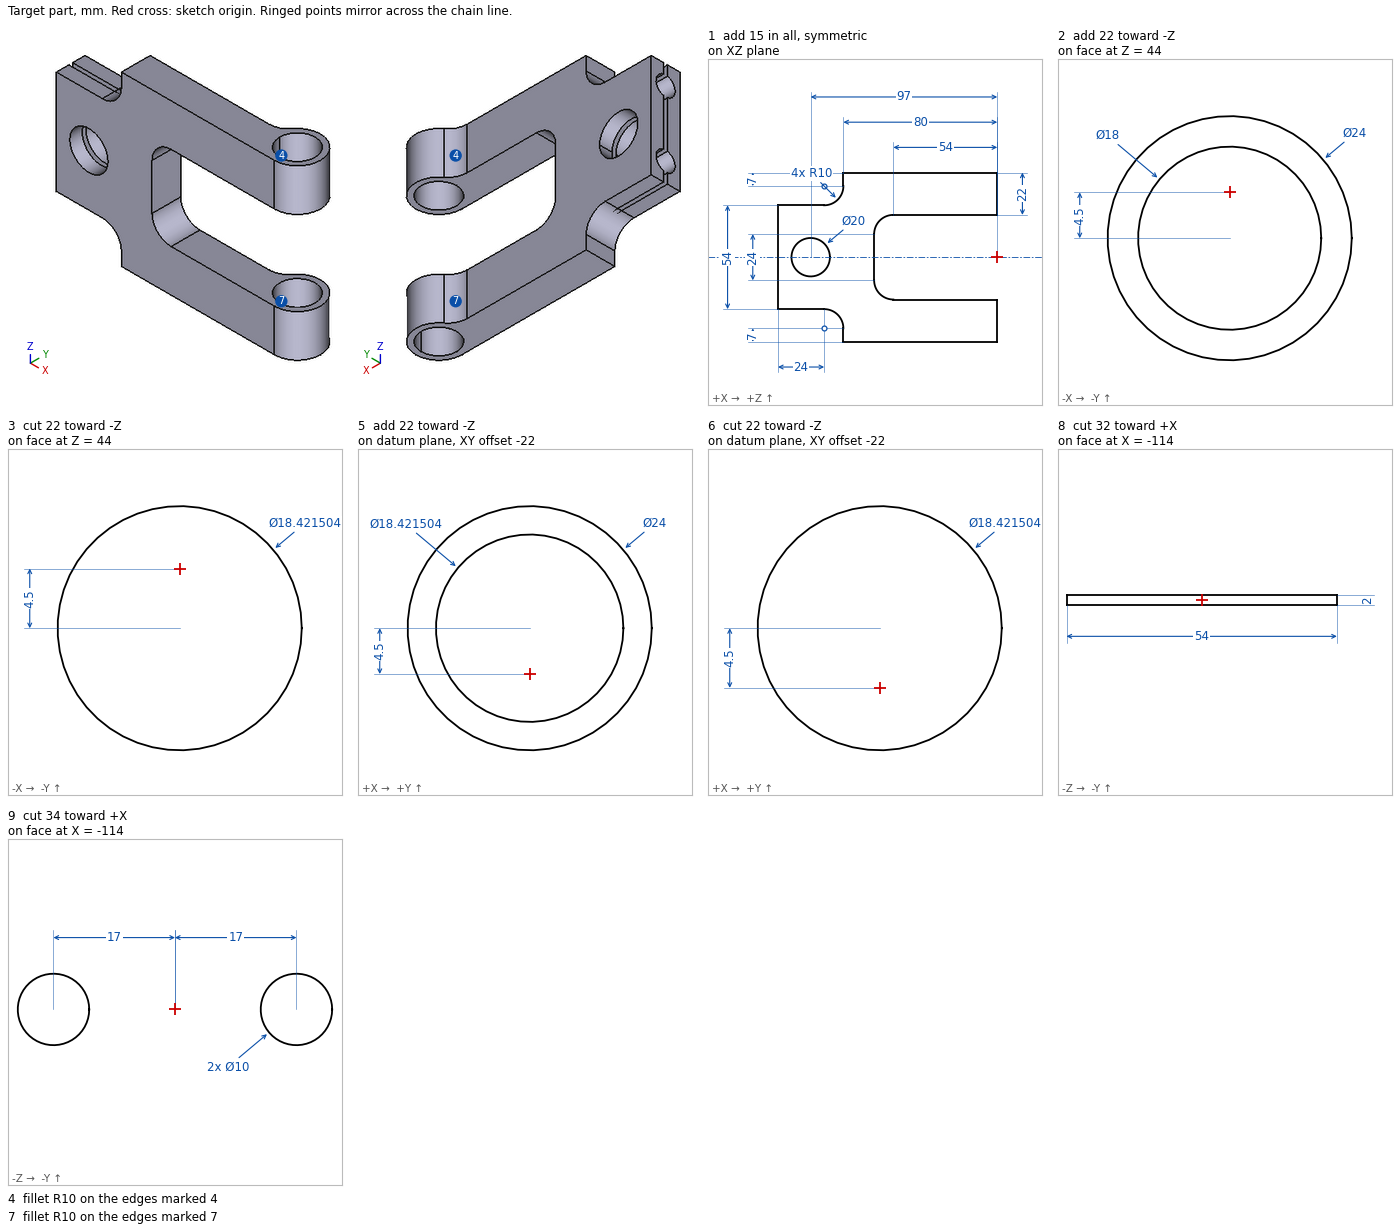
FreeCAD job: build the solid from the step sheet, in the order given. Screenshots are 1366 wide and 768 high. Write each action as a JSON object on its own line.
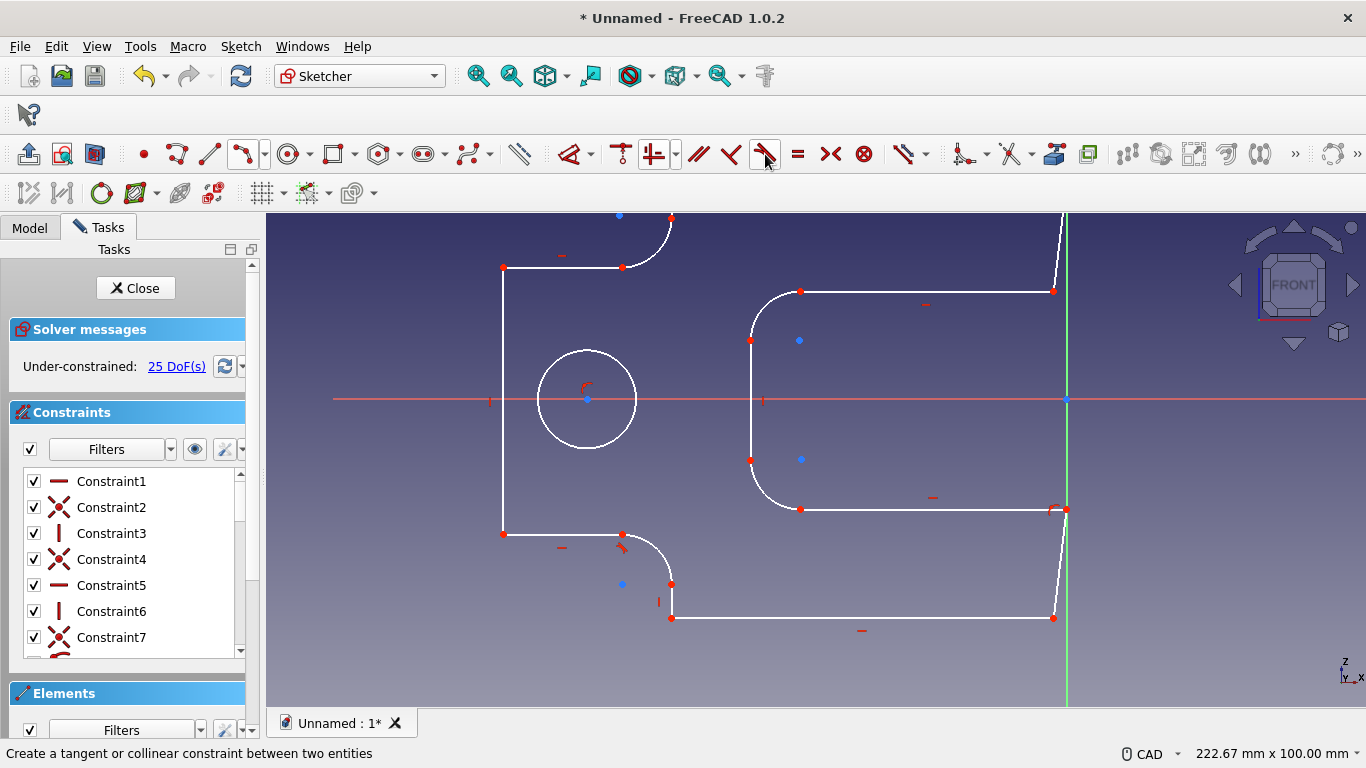
{"action": "left_click", "coordinate": [539, 268]}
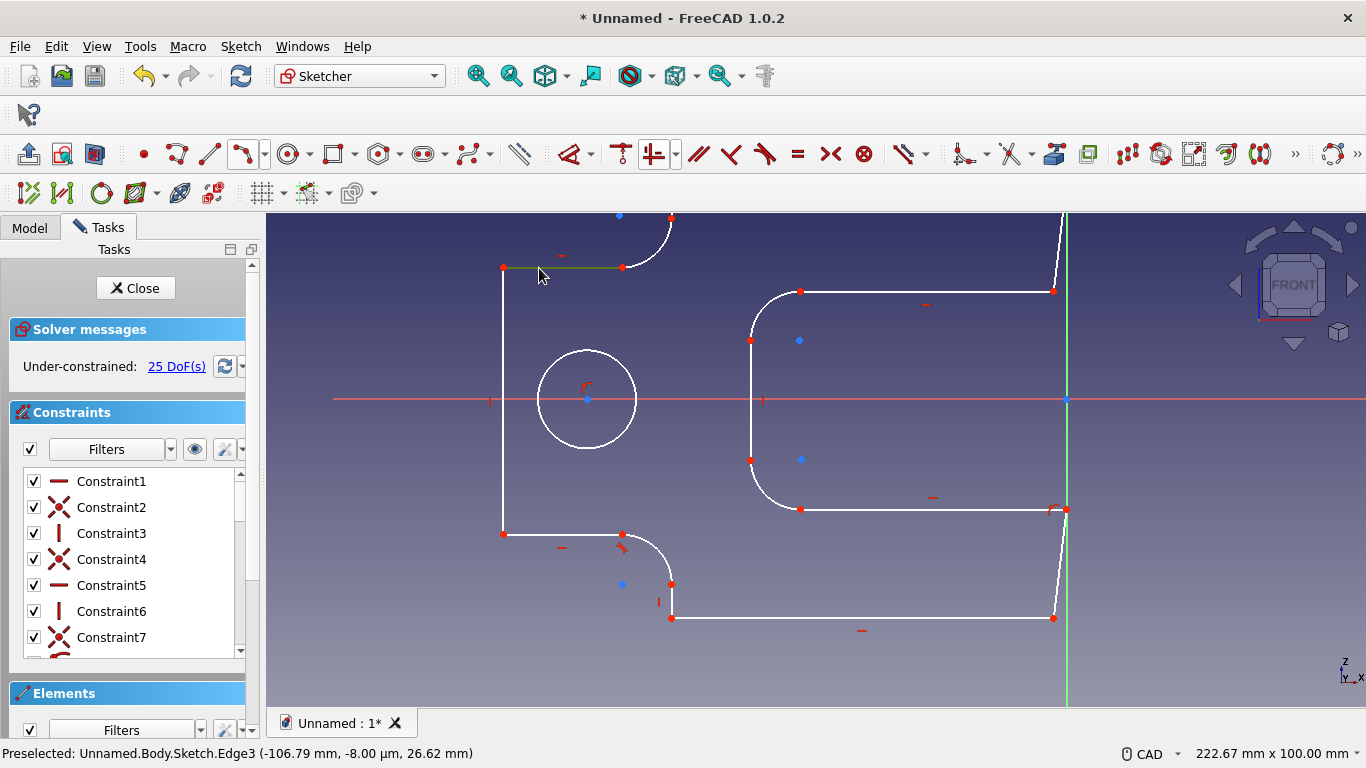
{"action": "left_click", "coordinate": [644, 262]}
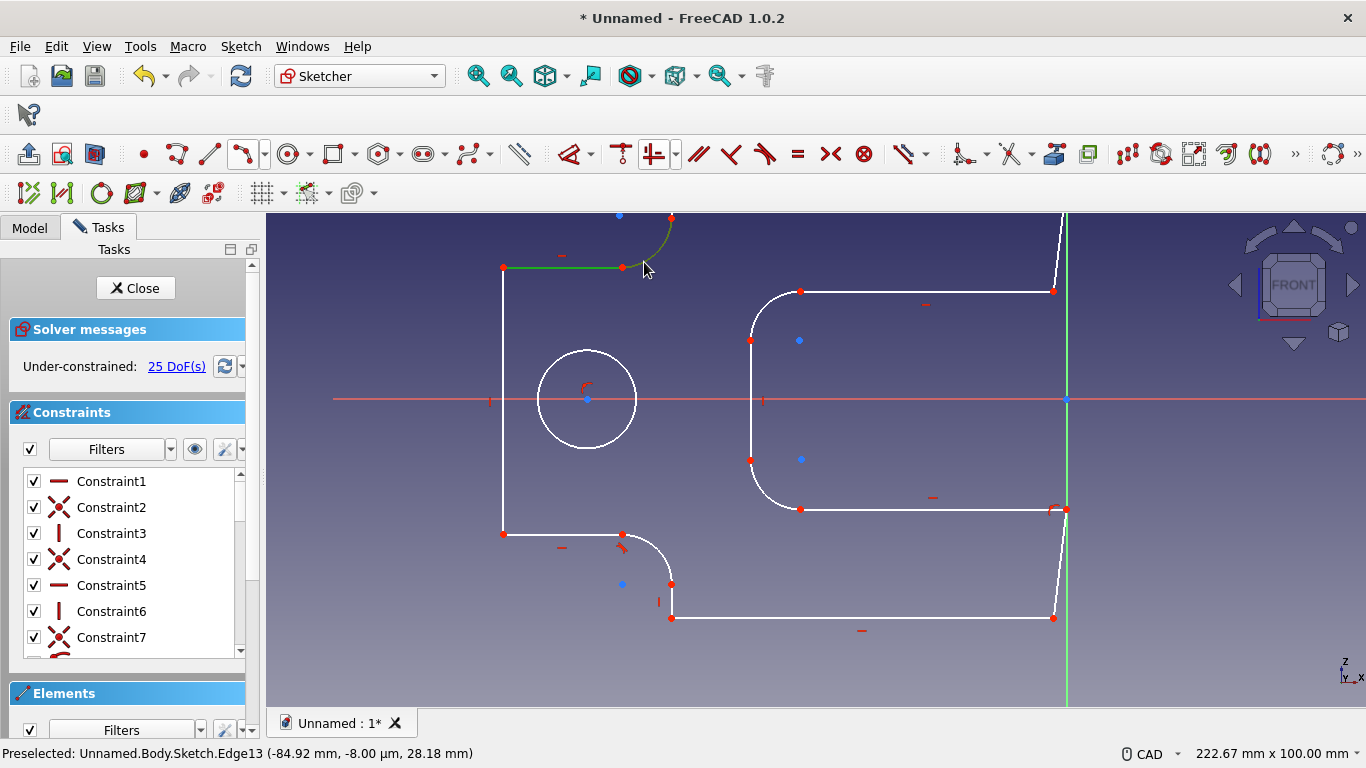
{"action": "left_click", "coordinate": [765, 154]}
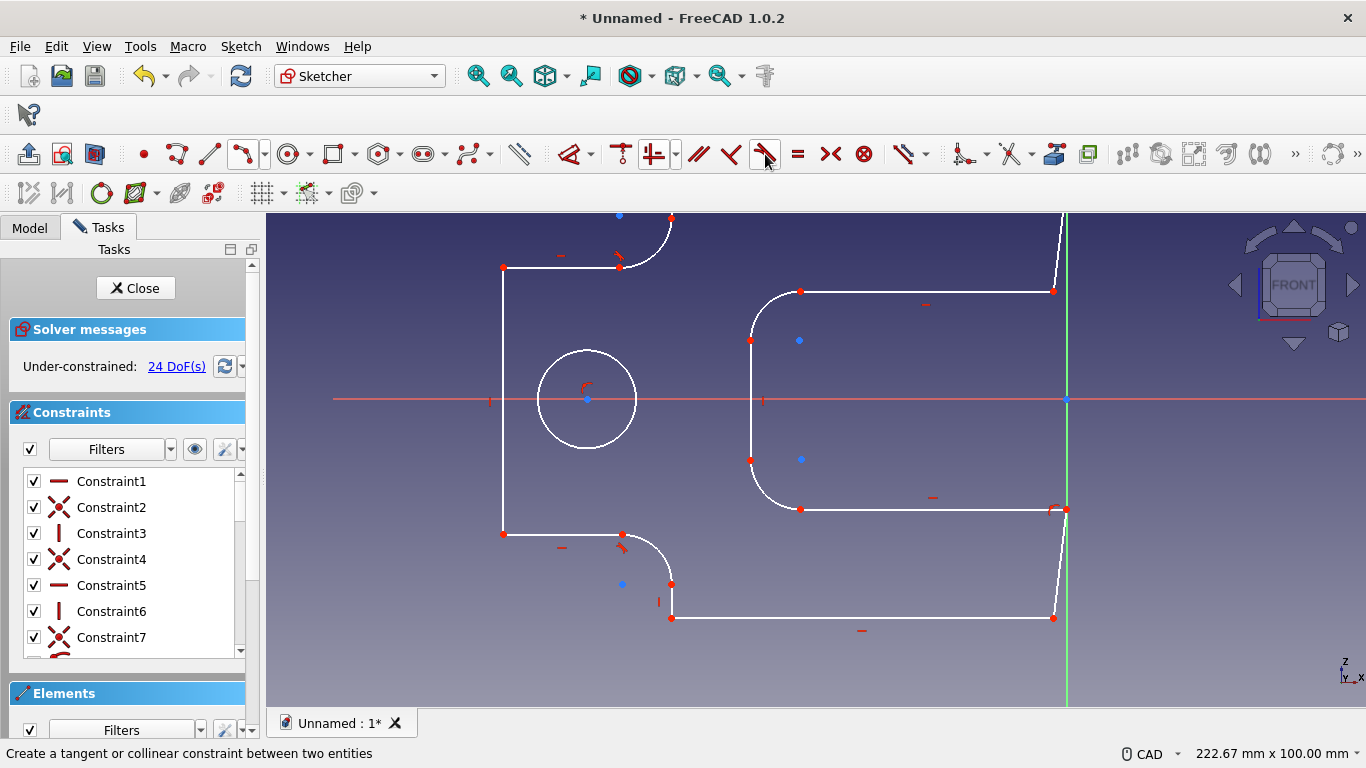
{"action": "scroll", "coordinate": [671, 583], "scroll_direction": "down", "scroll_amount": 2}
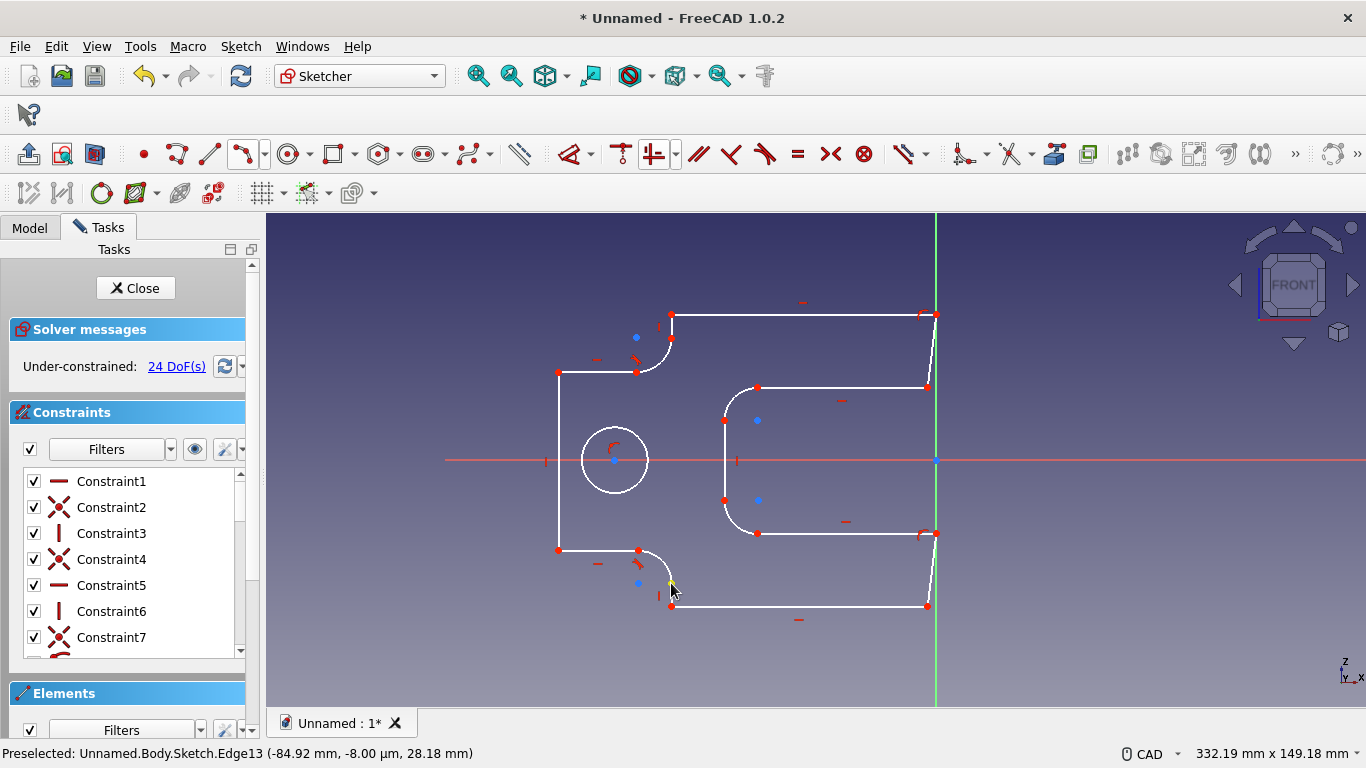
{"action": "scroll", "coordinate": [672, 332], "scroll_direction": "up", "scroll_amount": 4}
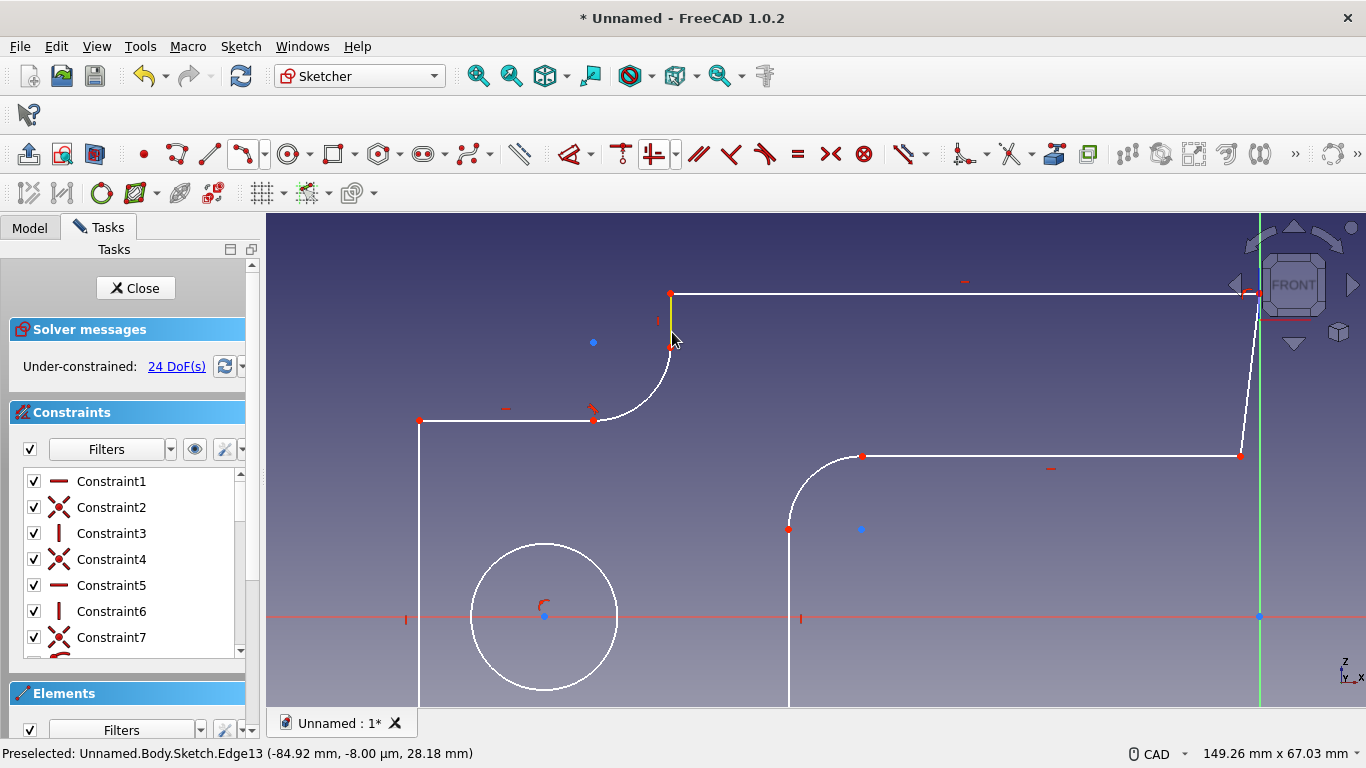
{"action": "left_click", "coordinate": [671, 331]}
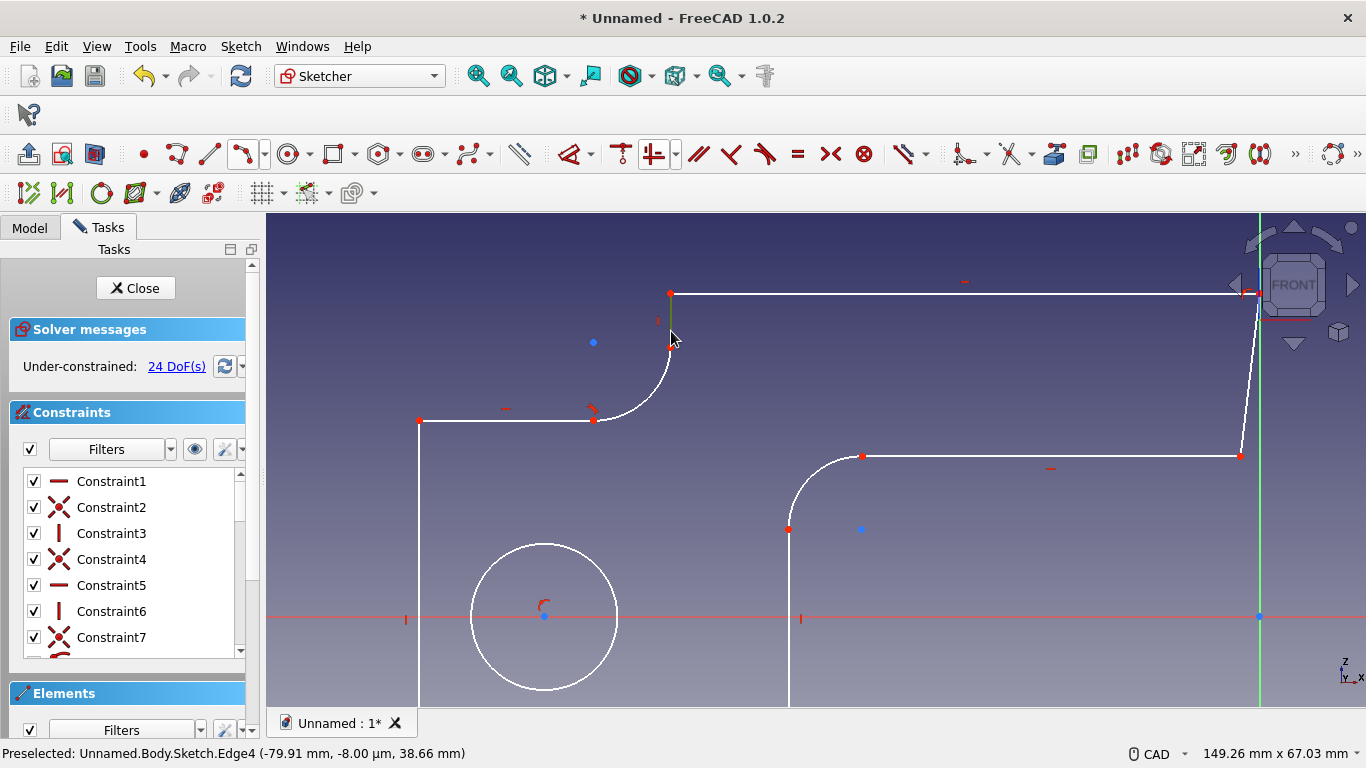
{"action": "left_click", "coordinate": [627, 413]}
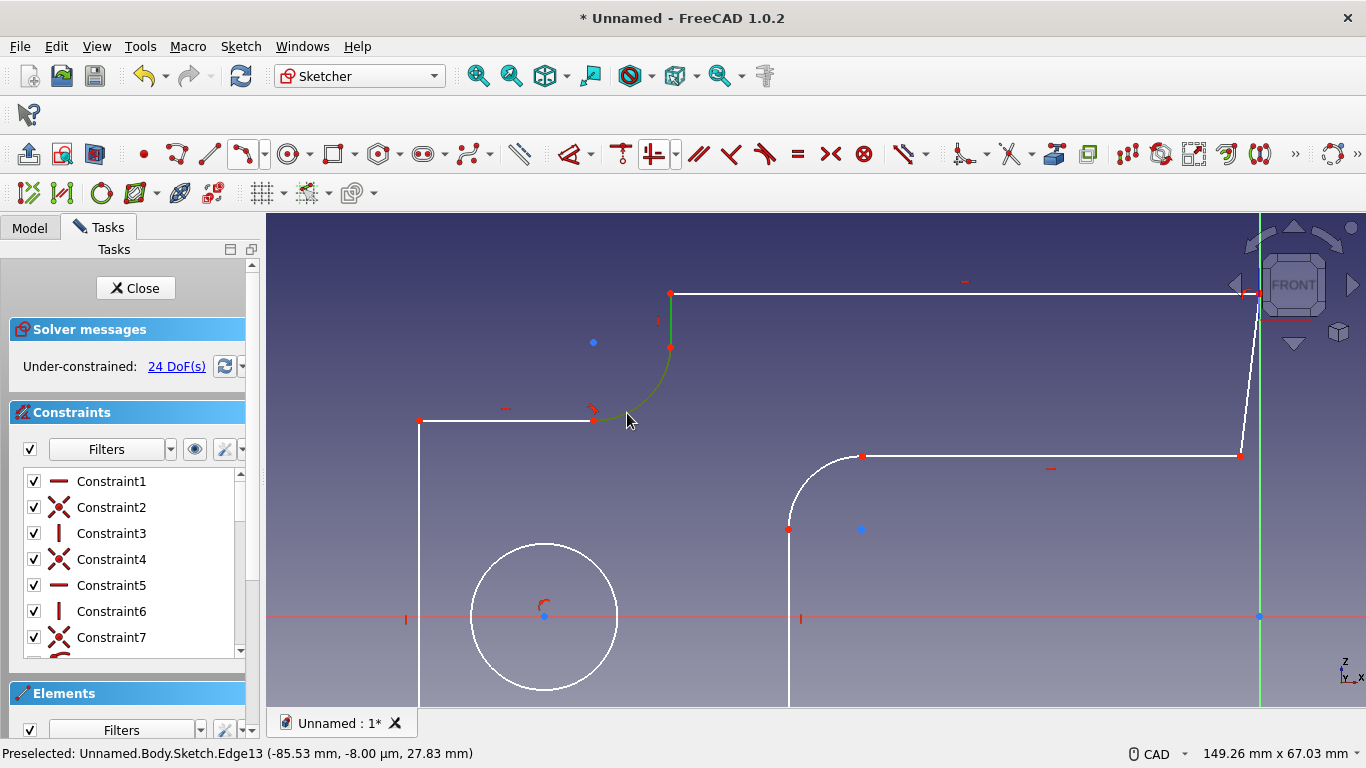
{"action": "left_click", "coordinate": [765, 154]}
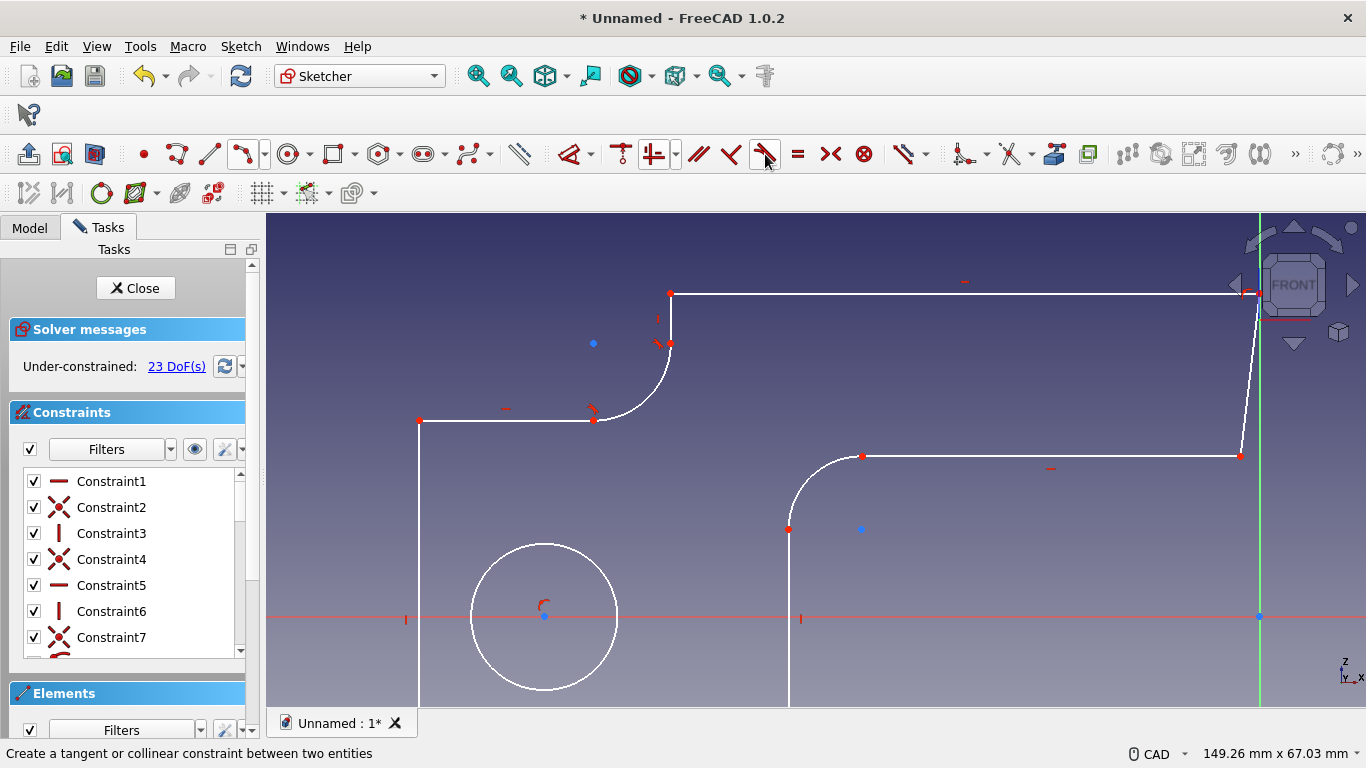
{"action": "left_click", "coordinate": [1127, 456]}